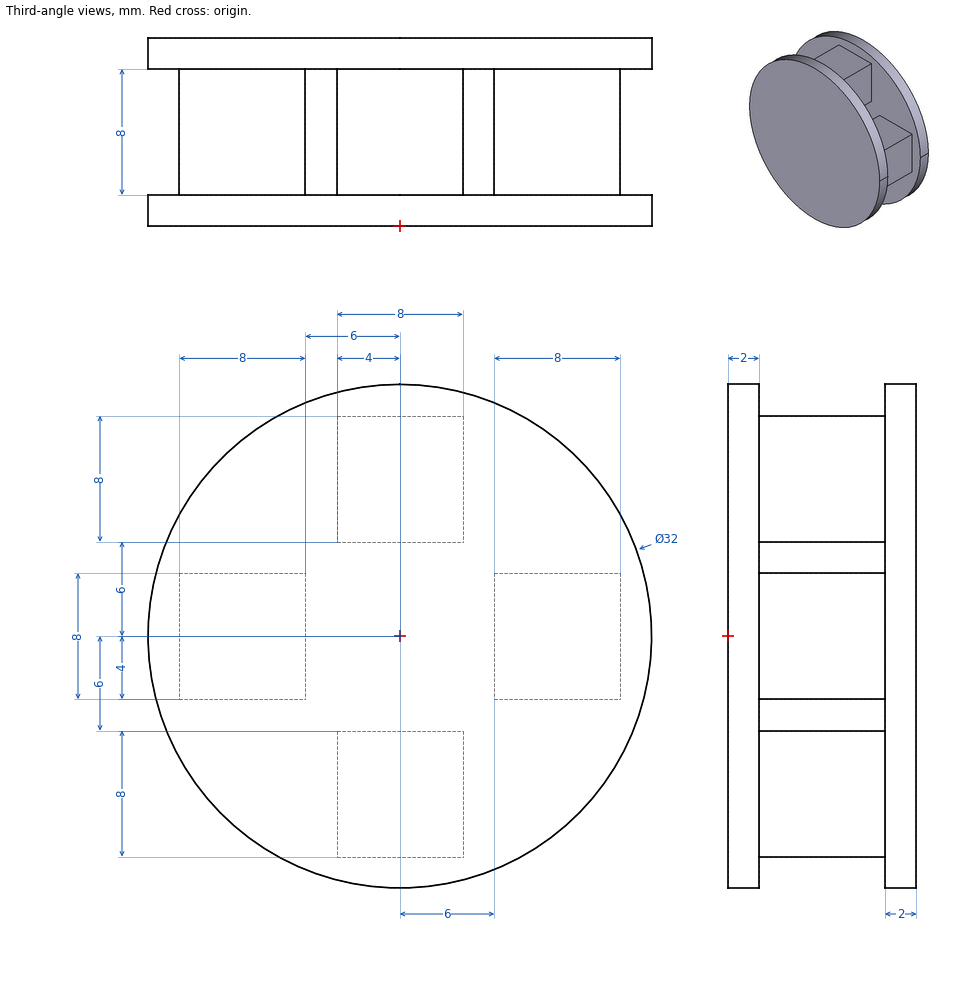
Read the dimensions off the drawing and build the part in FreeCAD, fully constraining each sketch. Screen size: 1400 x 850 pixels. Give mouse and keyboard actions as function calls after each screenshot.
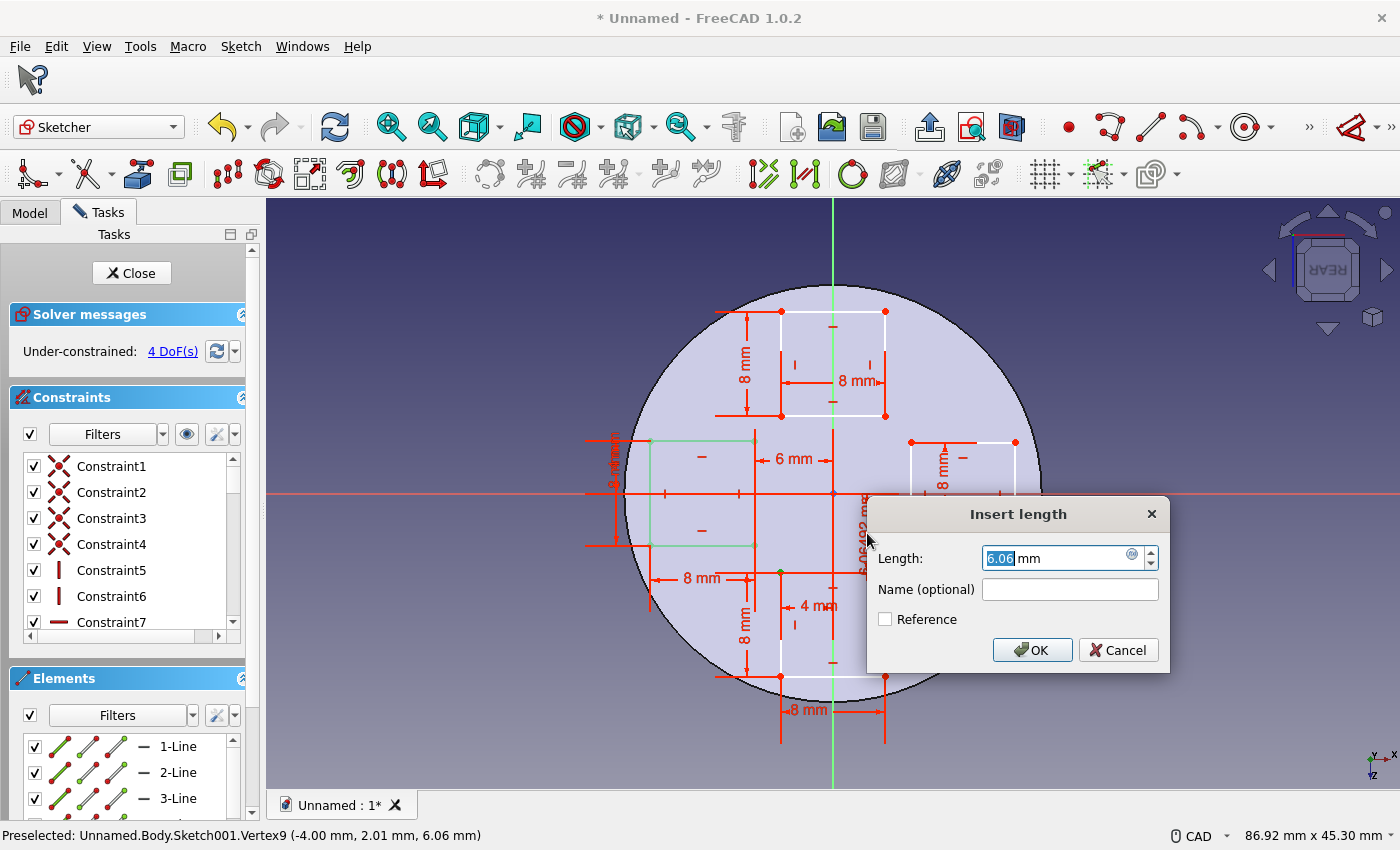
text(6)
key(Return)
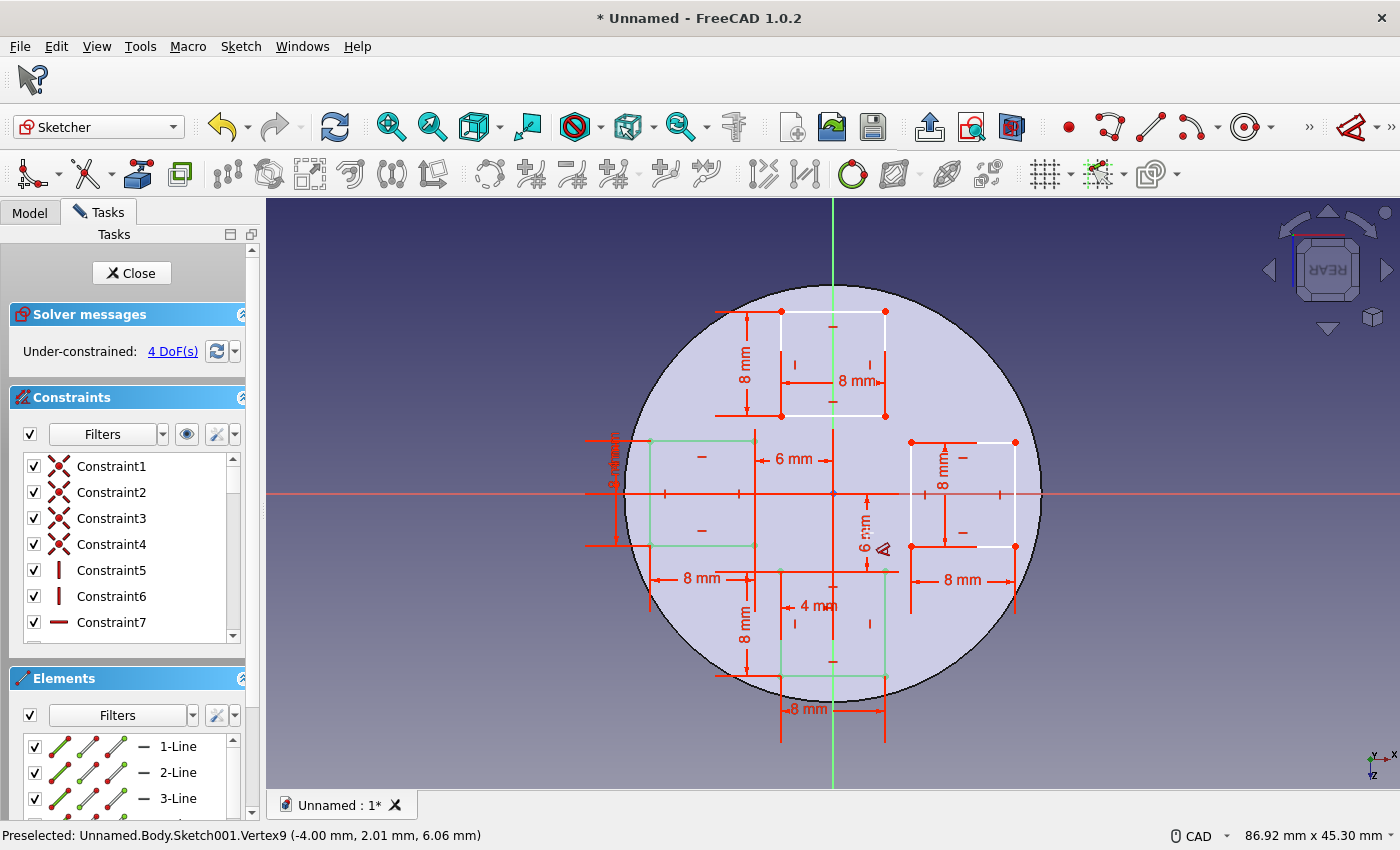
click(781, 312)
click(807, 278)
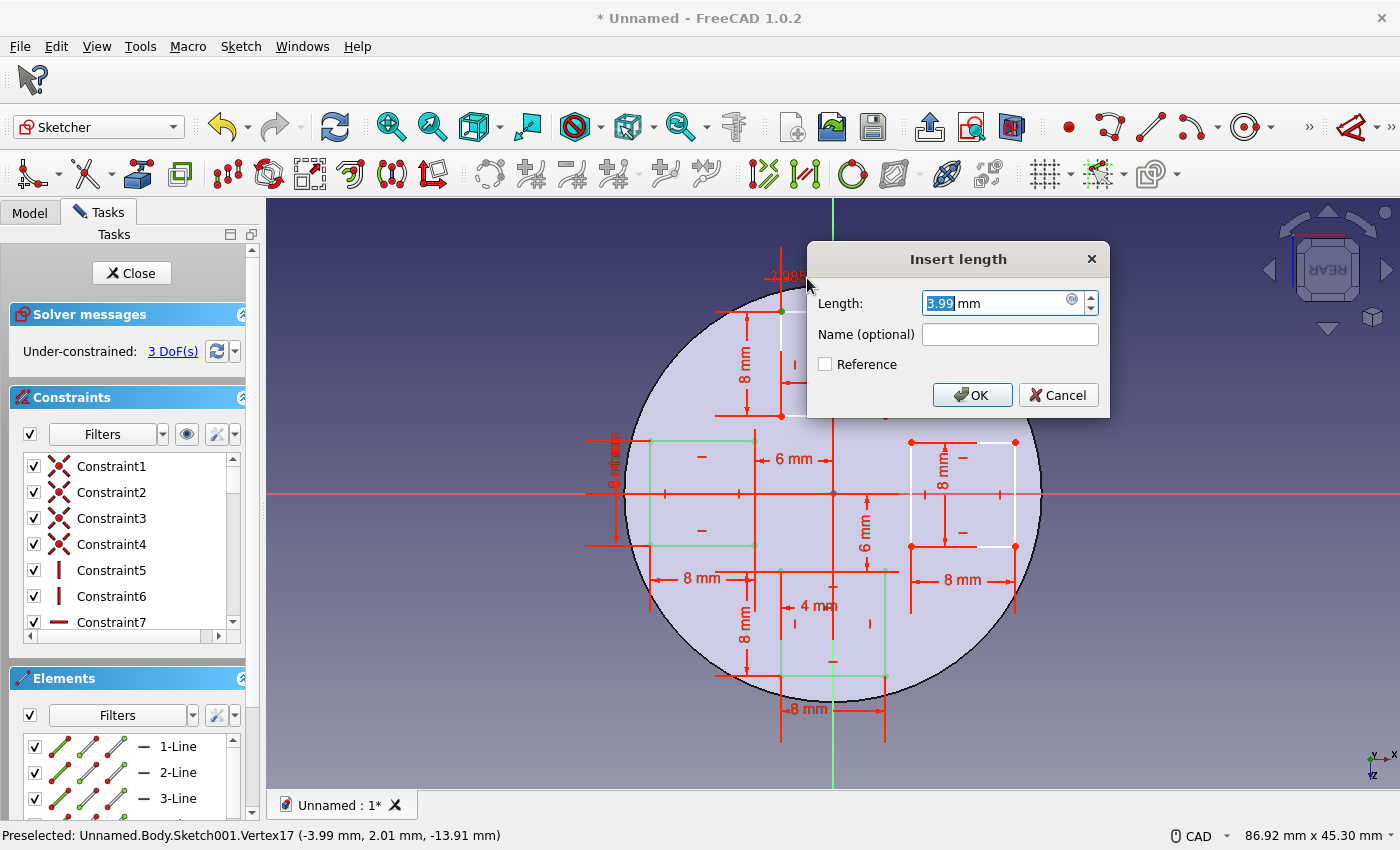
text(4)
key(Return)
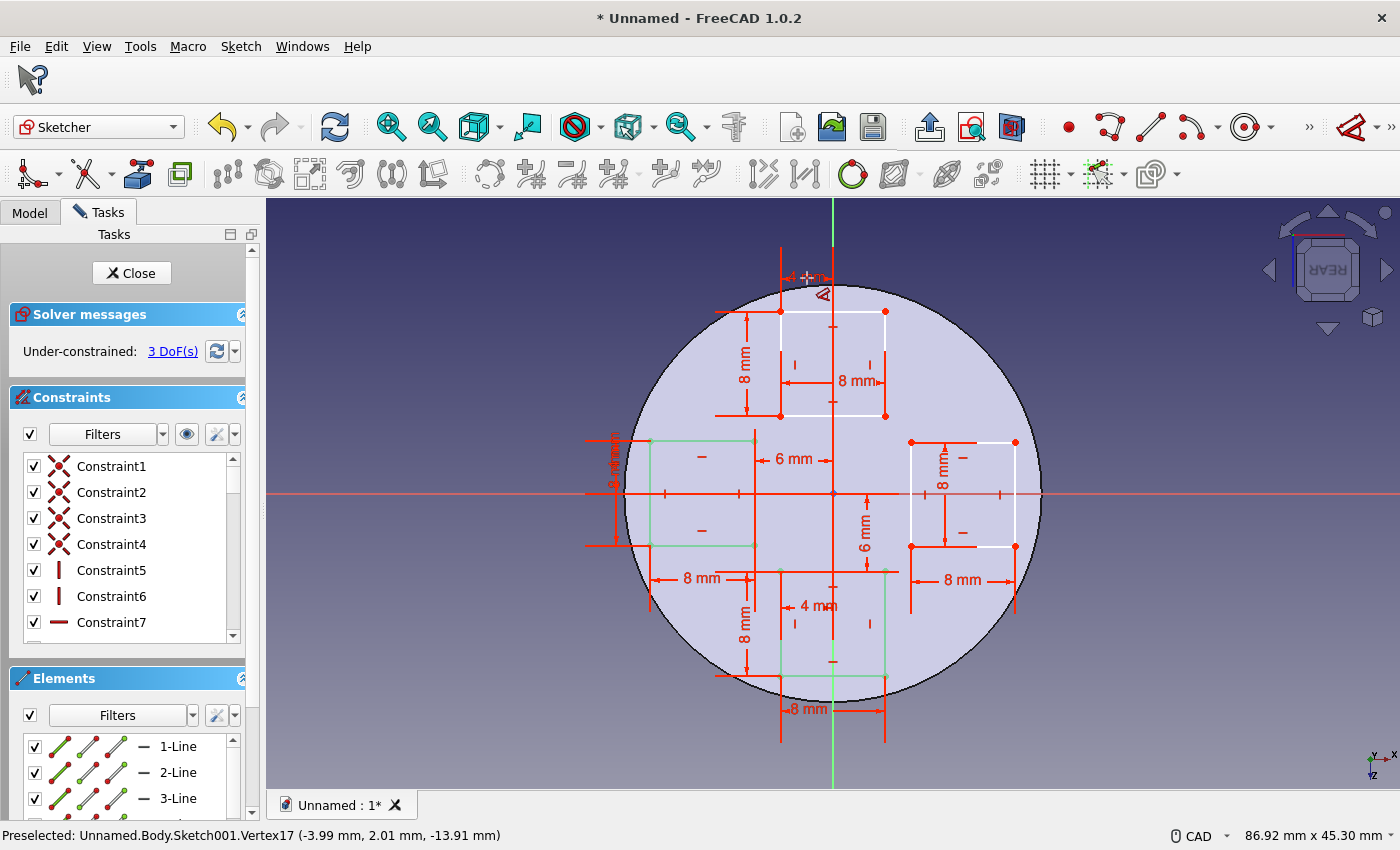
click(781, 416)
click(747, 428)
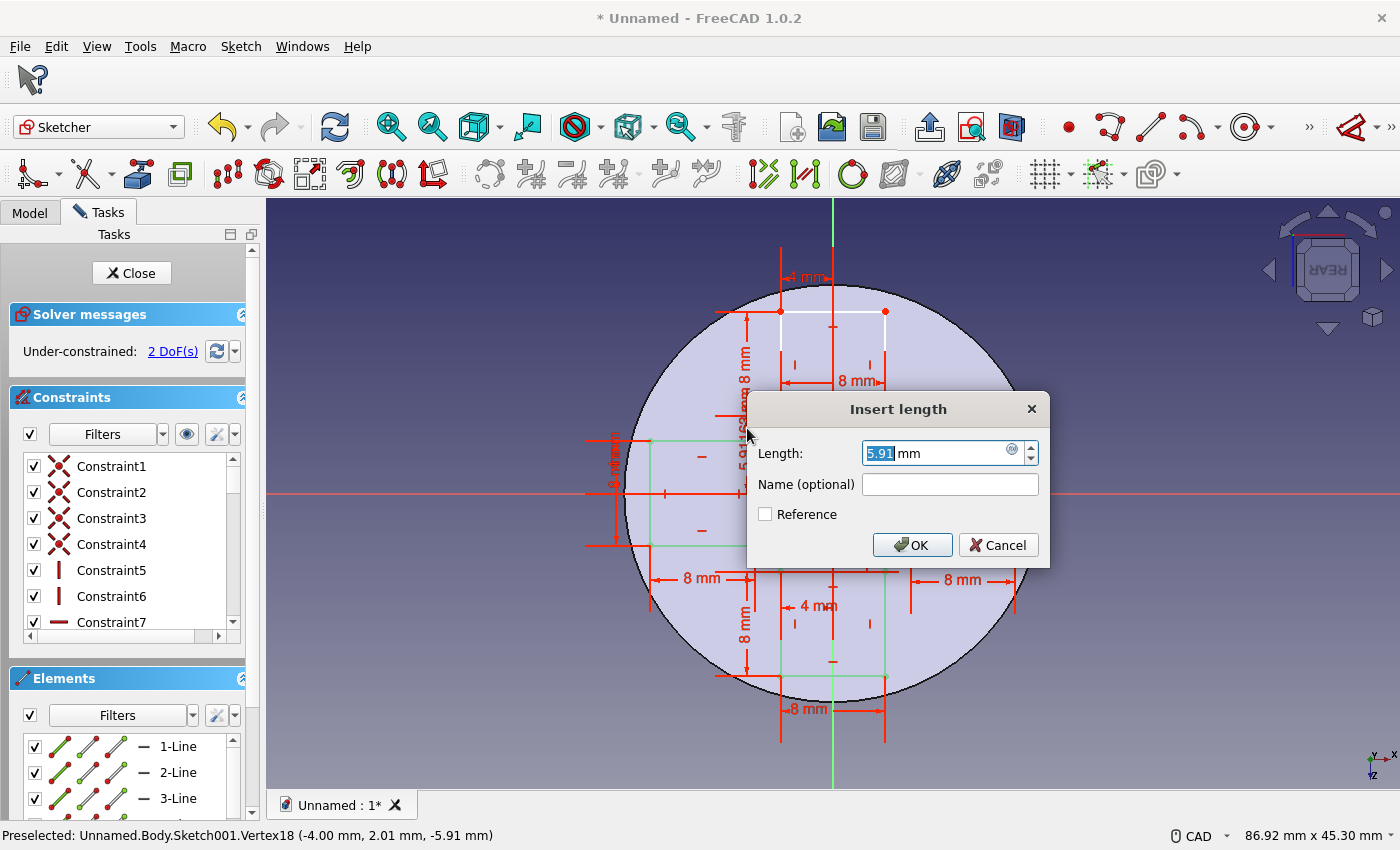
text(6)
key(Return)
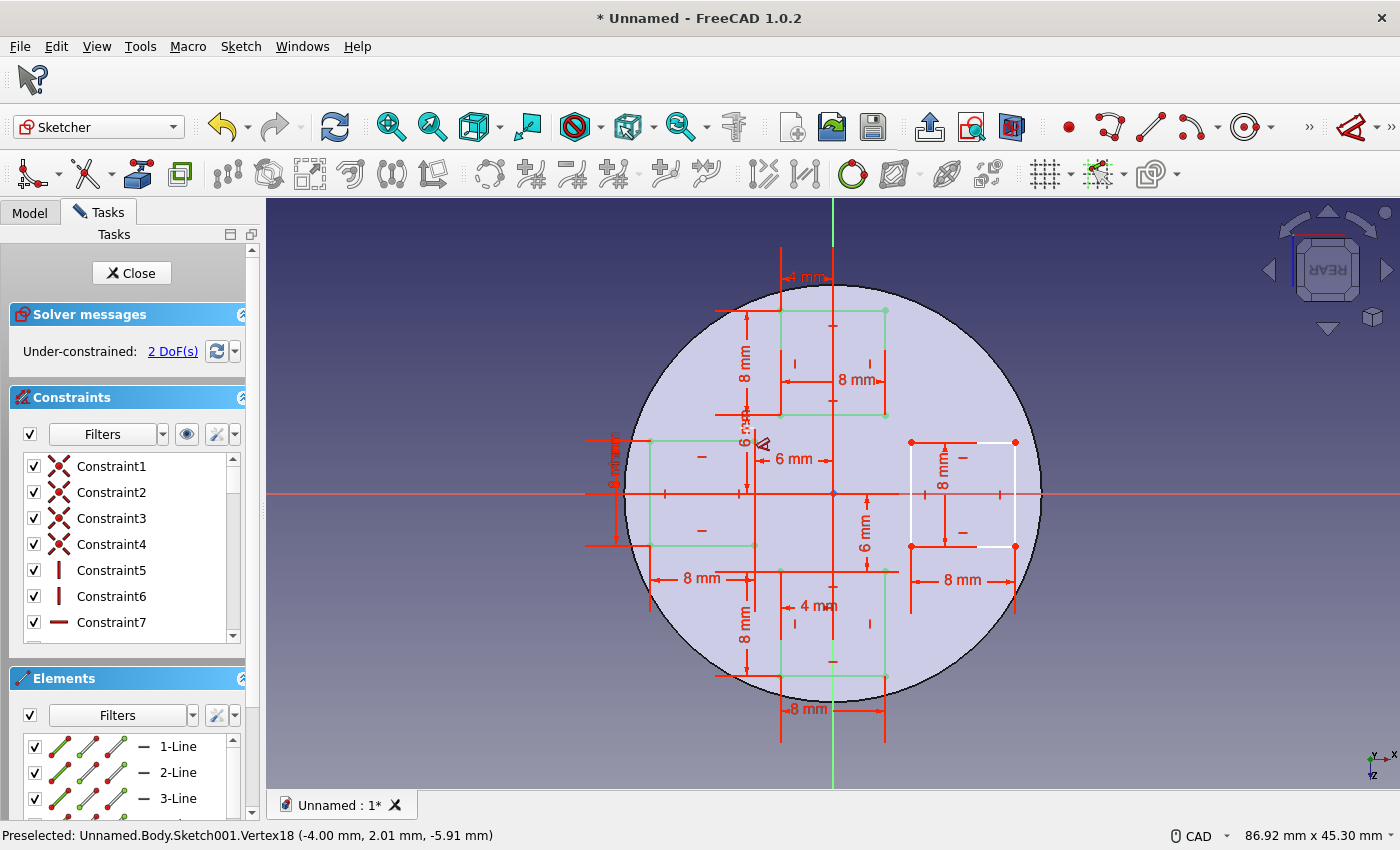
click(911, 443)
click(899, 409)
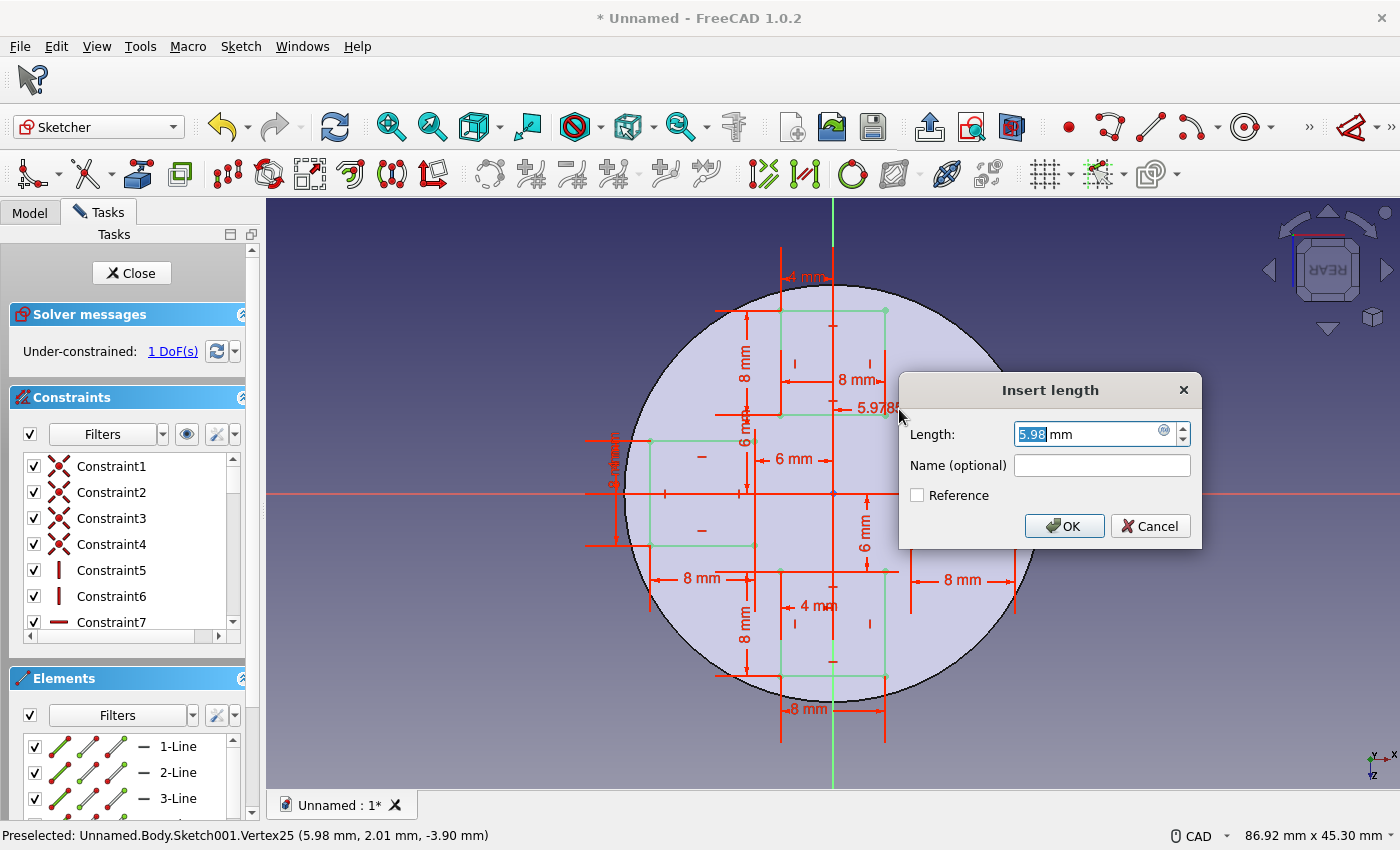
text(6)
key(Return)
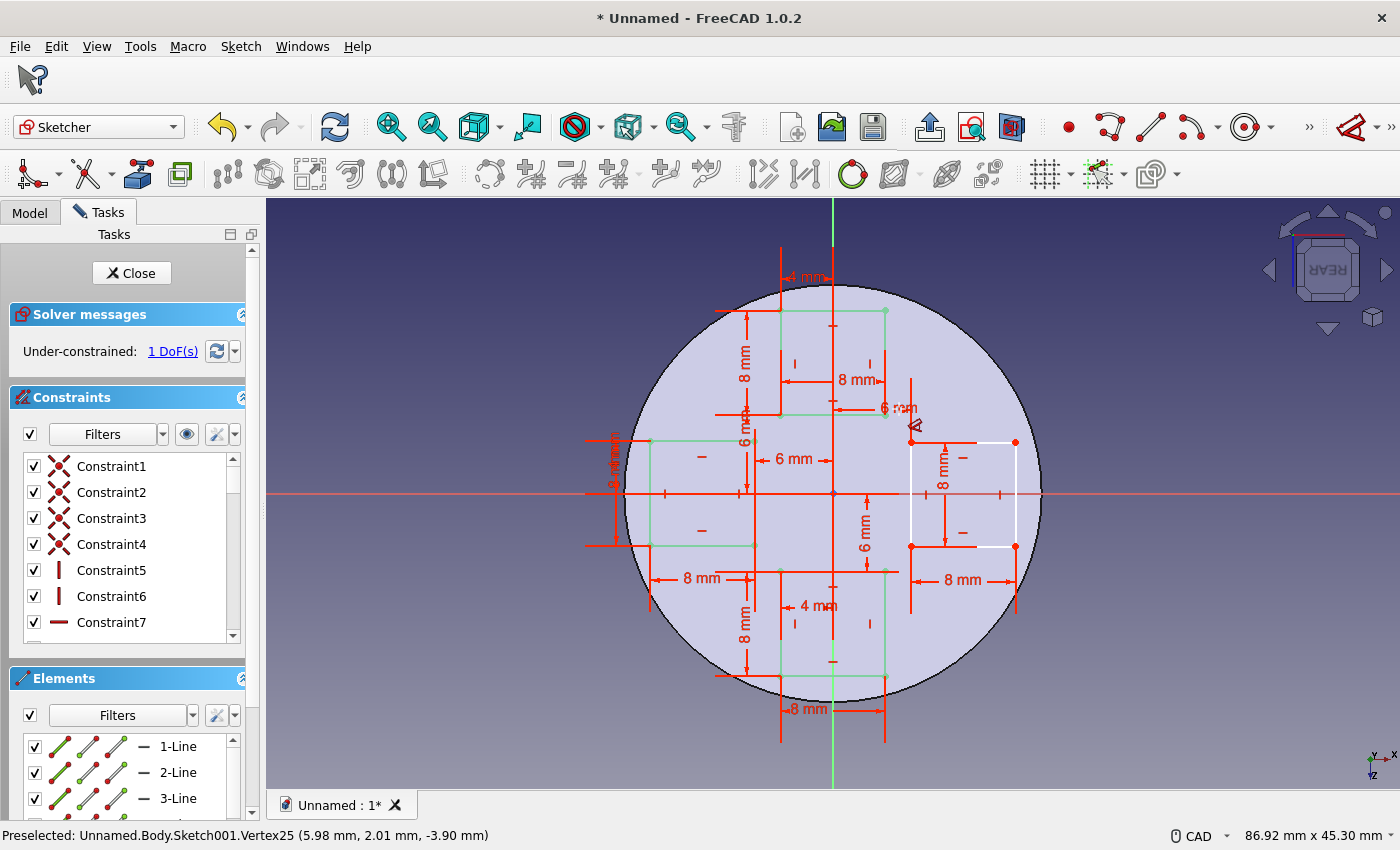
click(911, 443)
click(799, 480)